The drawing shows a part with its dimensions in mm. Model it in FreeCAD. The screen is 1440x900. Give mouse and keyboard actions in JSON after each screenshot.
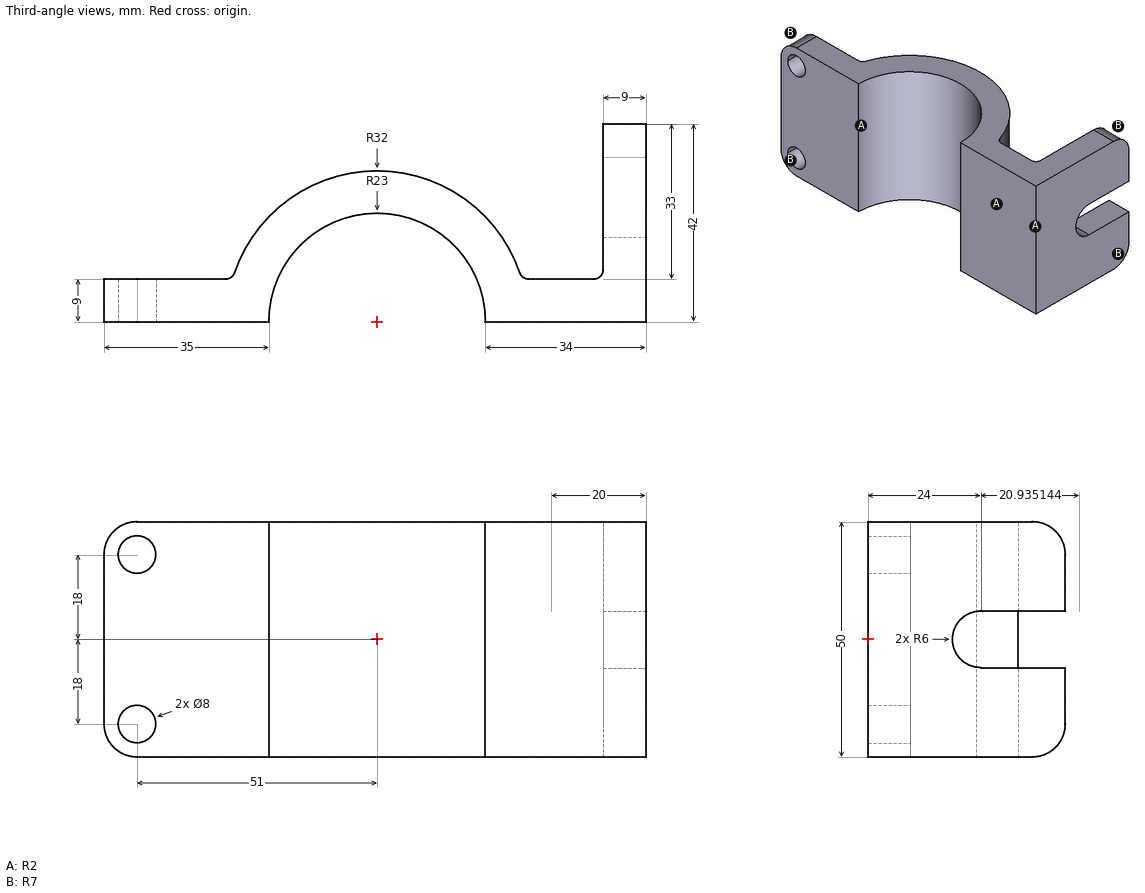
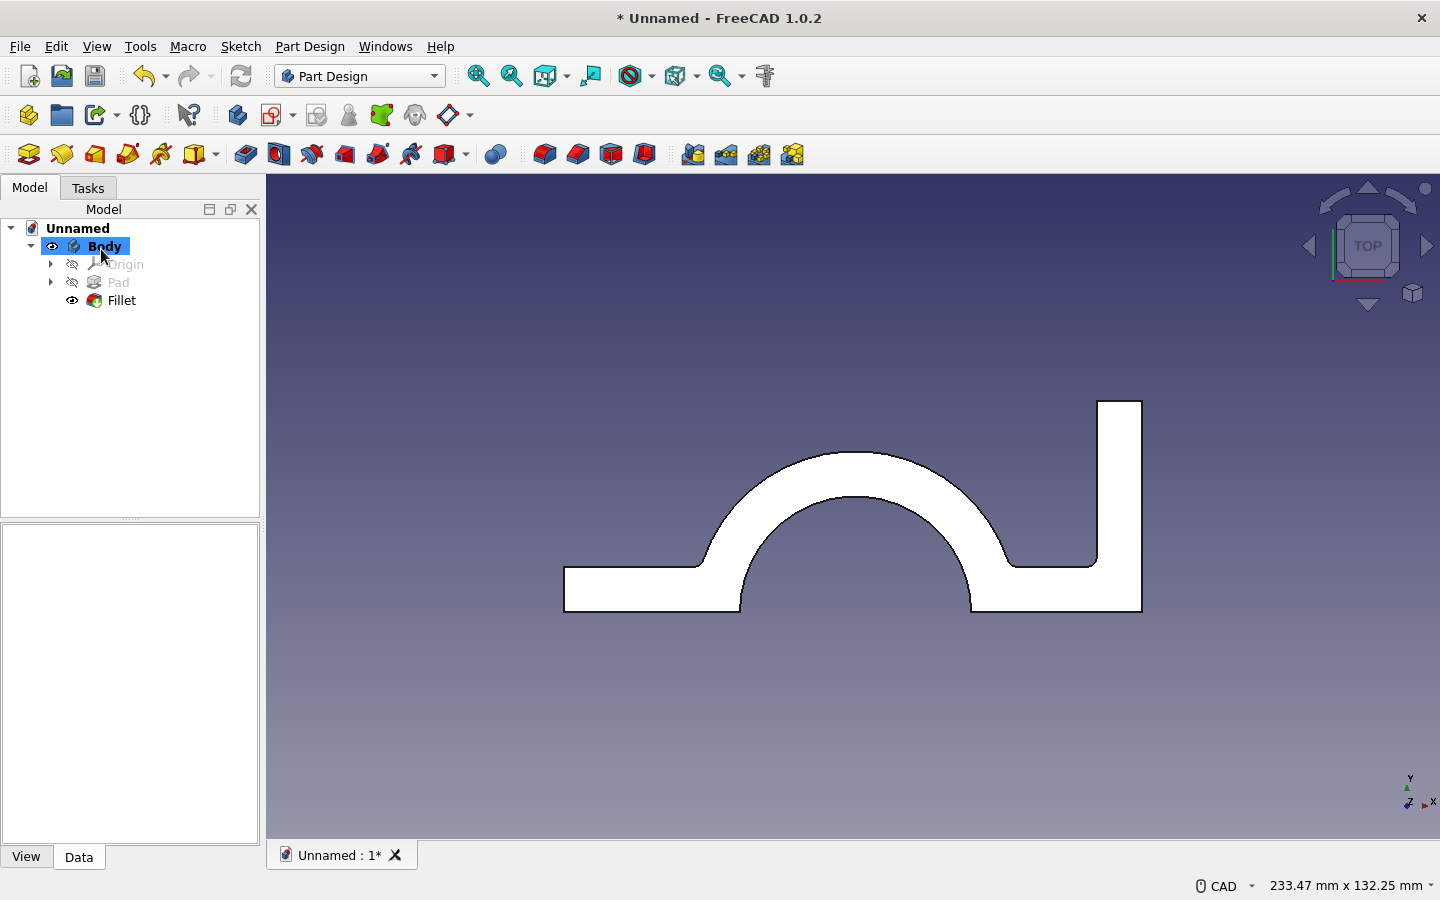
{"action": "left_click", "coordinate": [1120, 400]}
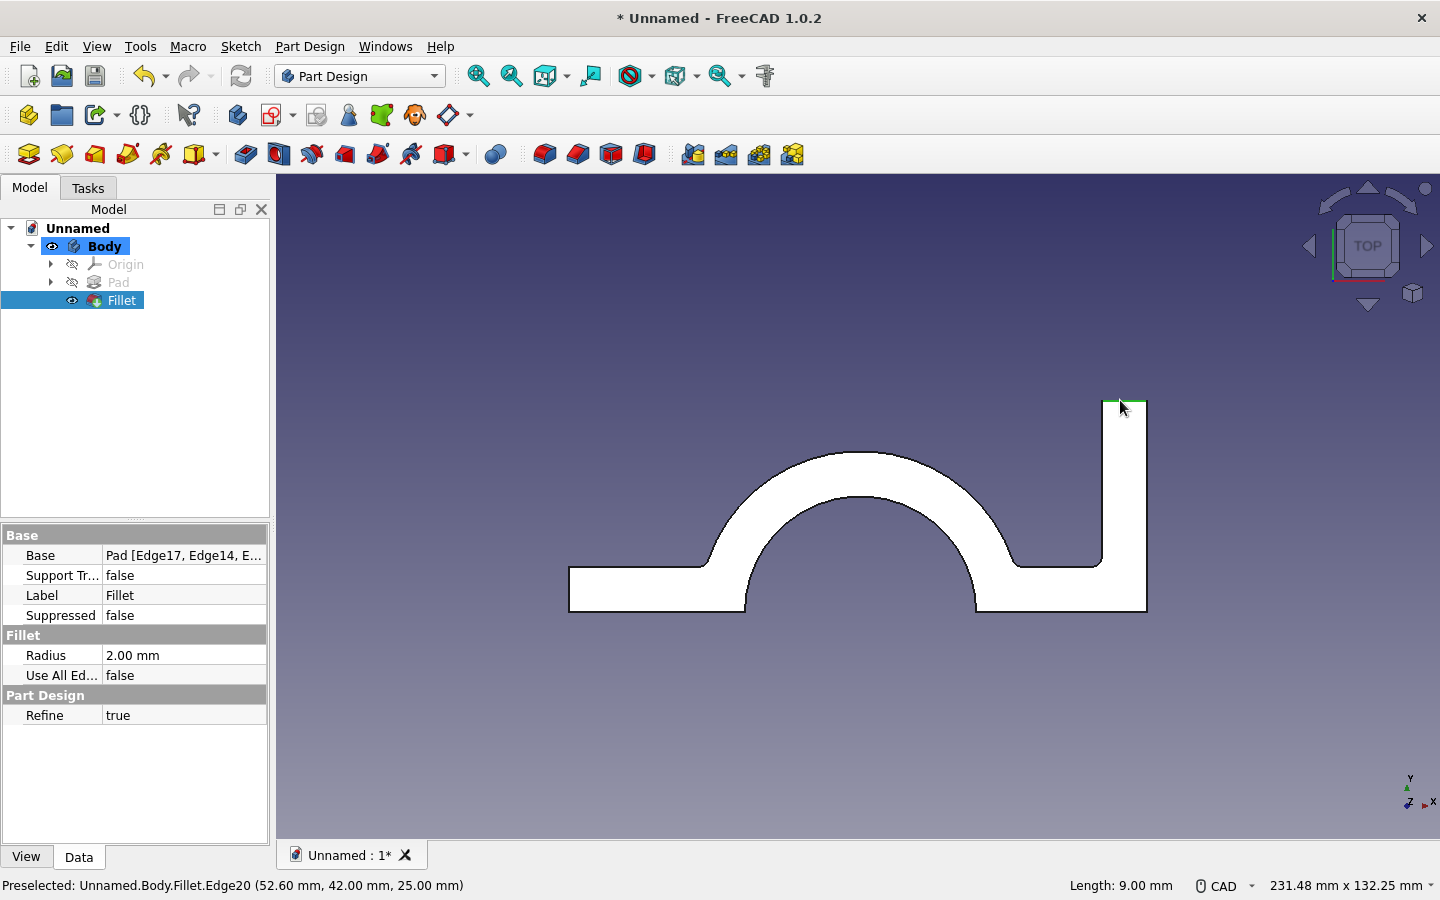
{"action": "left_click", "coordinate": [569, 588], "text": "ctrl"}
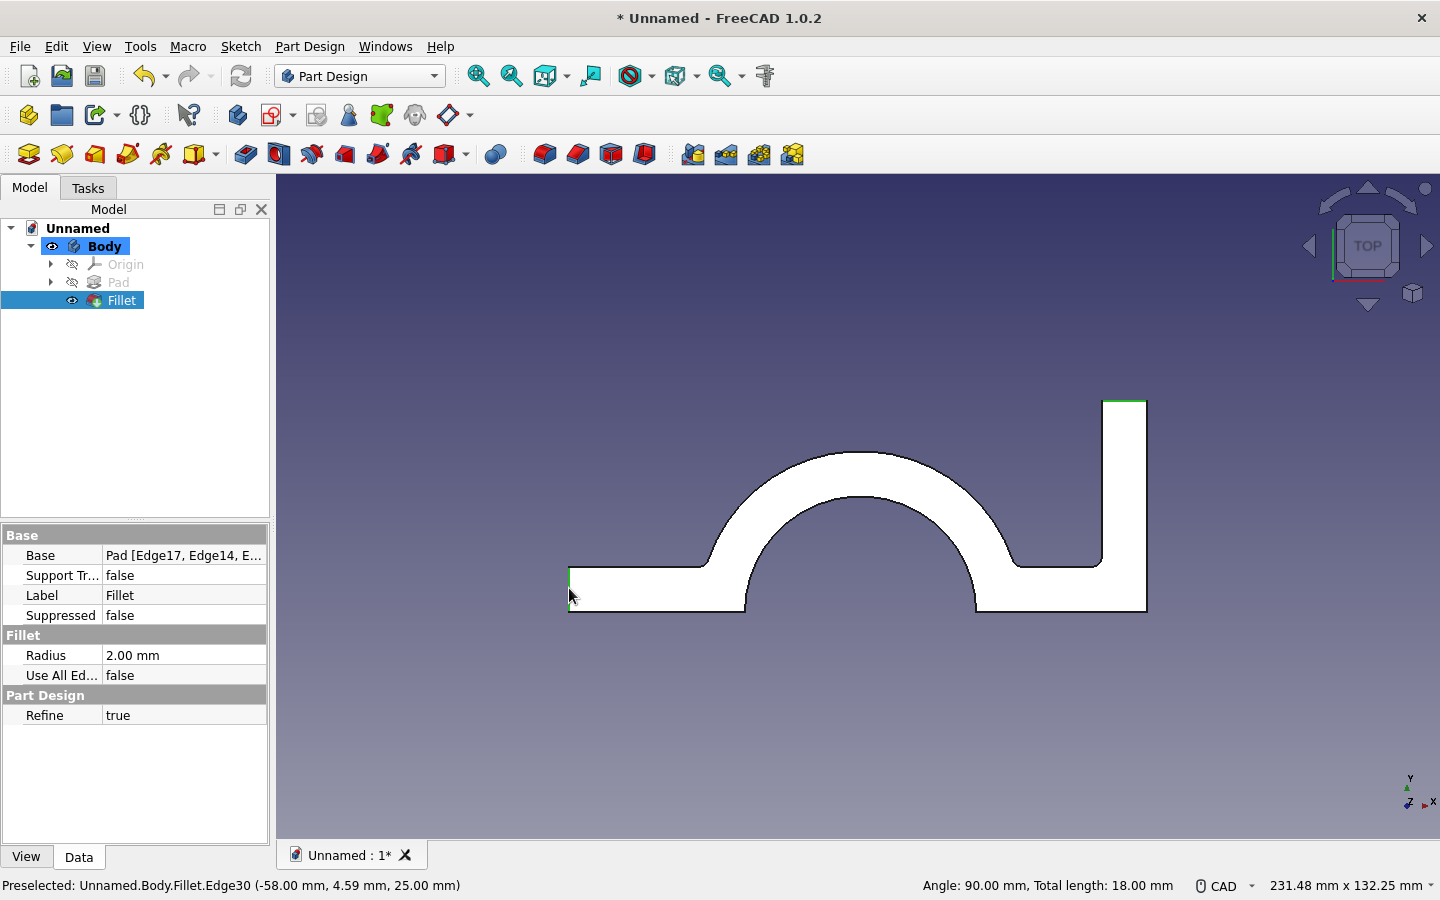
{"action": "key", "text": "0"}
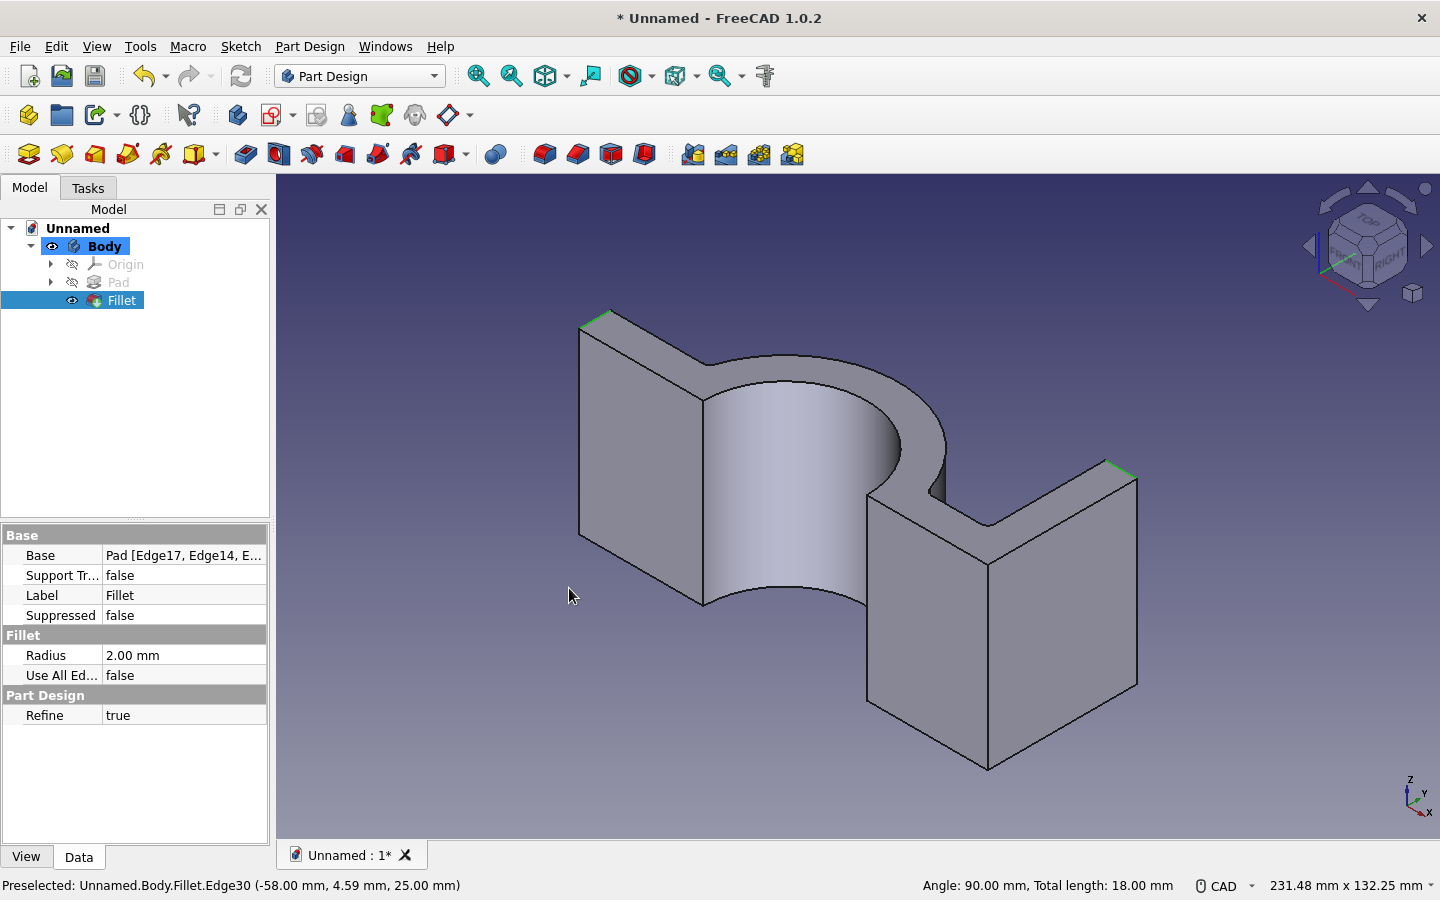
{"action": "key", "text": "1"}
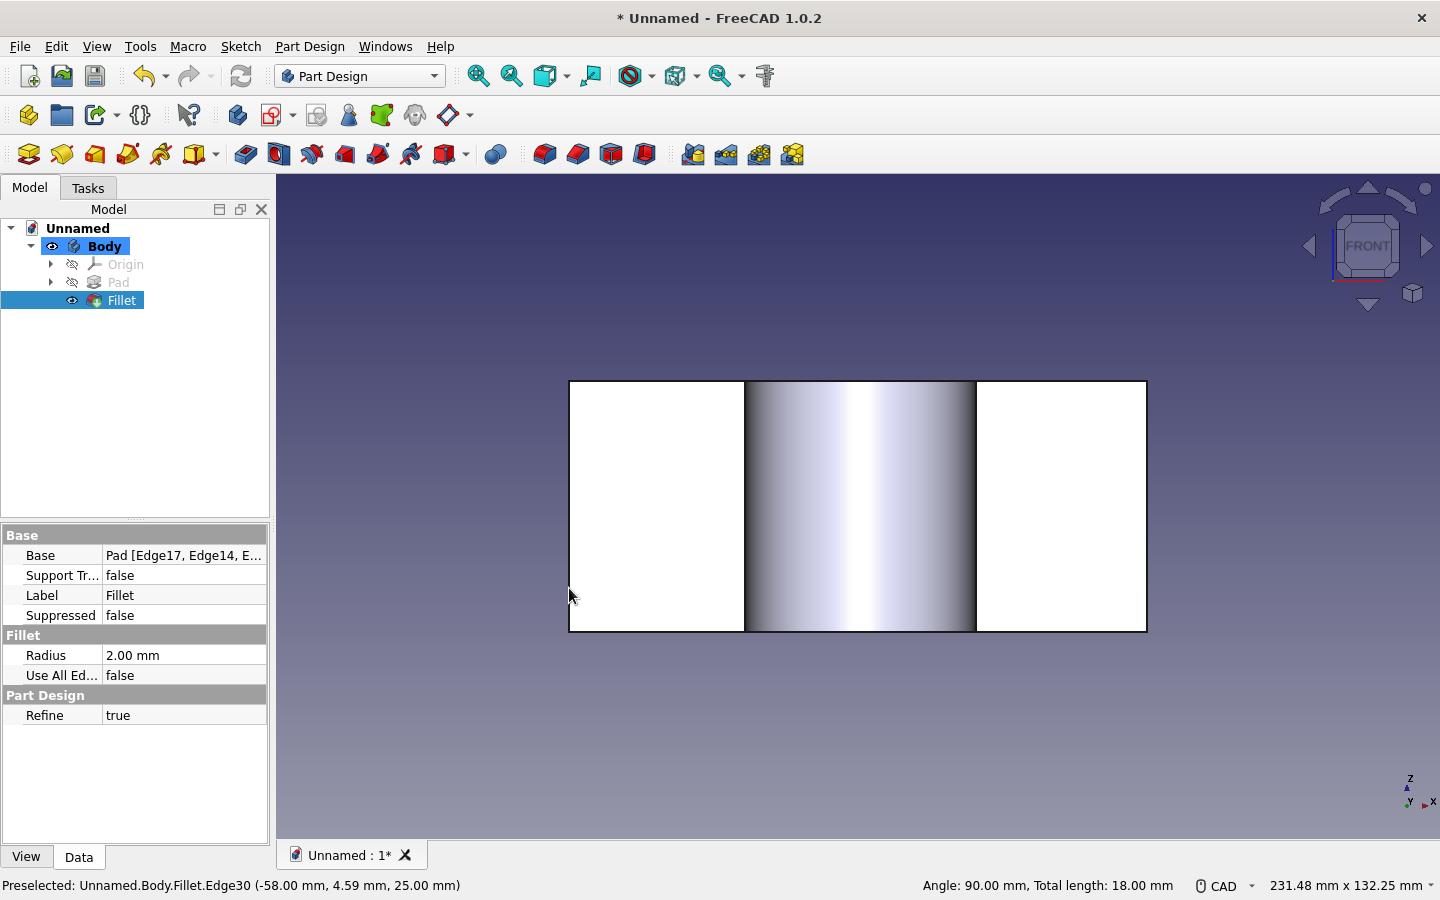
{"action": "key", "text": "3"}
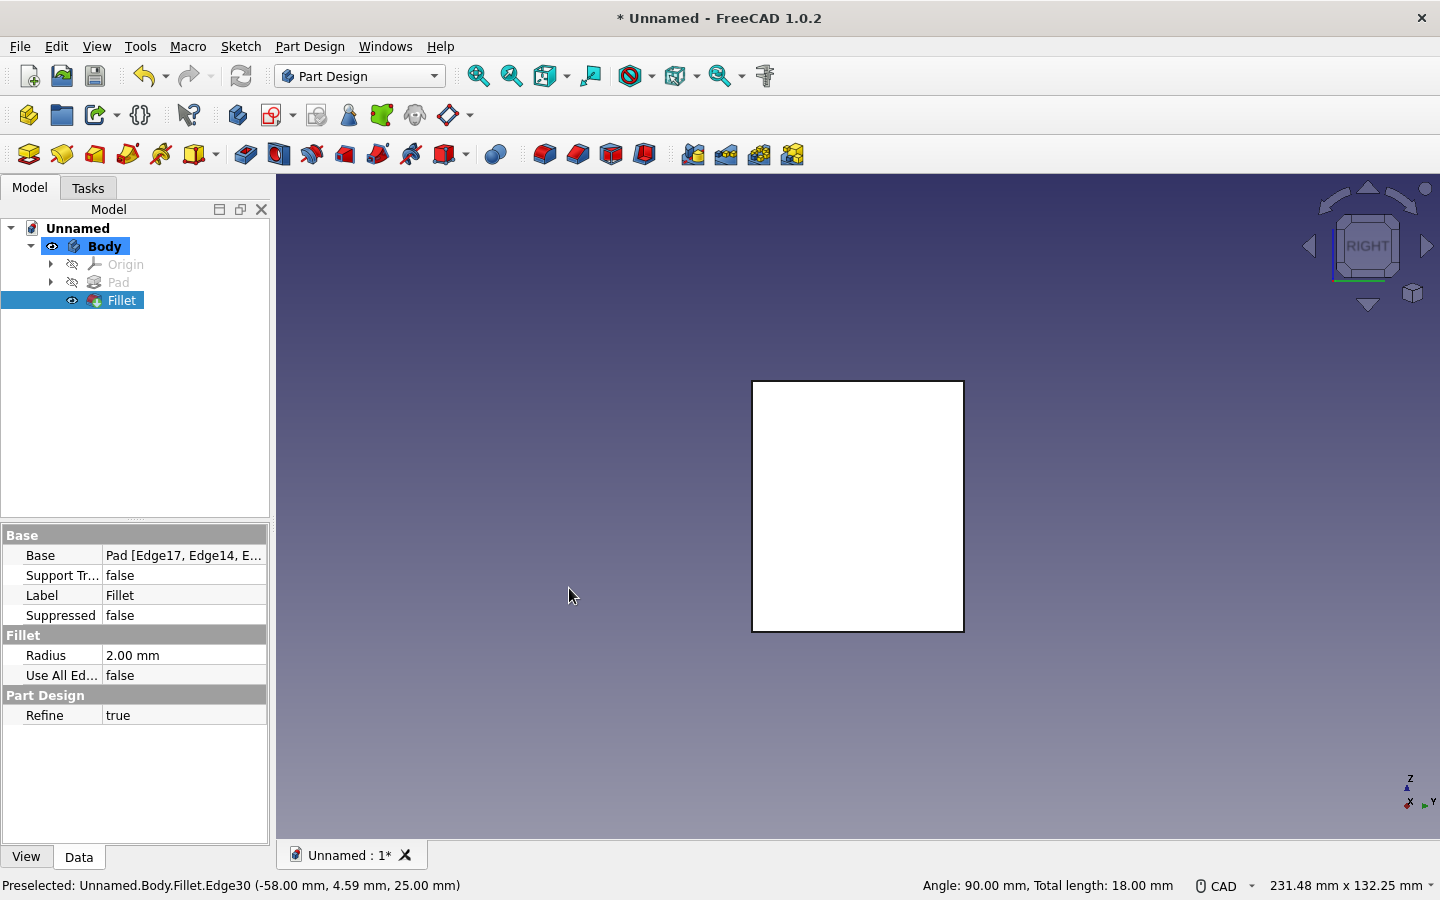
{"action": "left_click", "coordinate": [479, 76]}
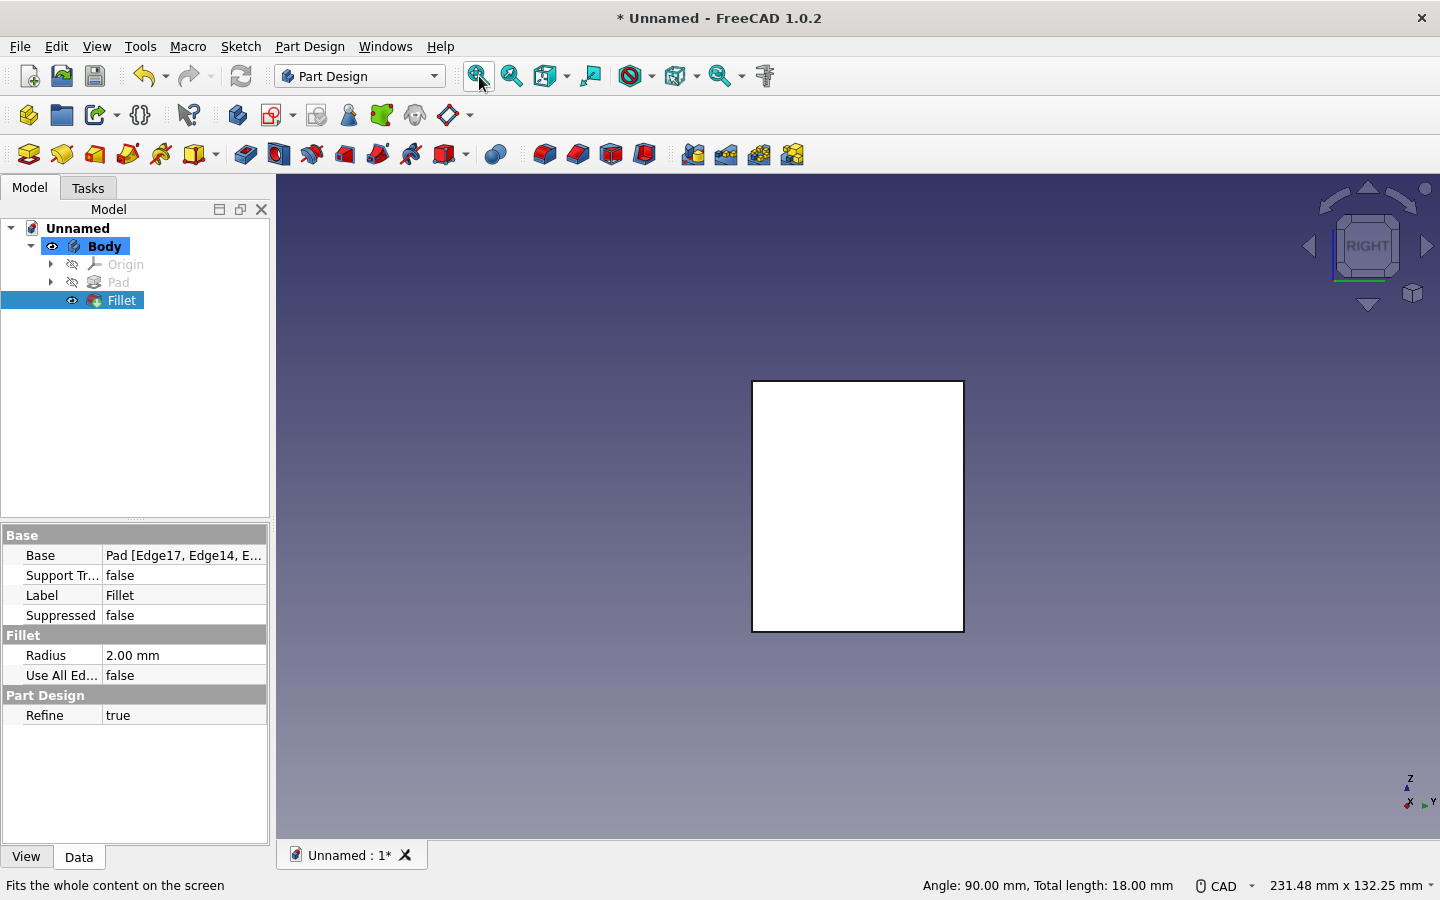
{"action": "key", "text": "5"}